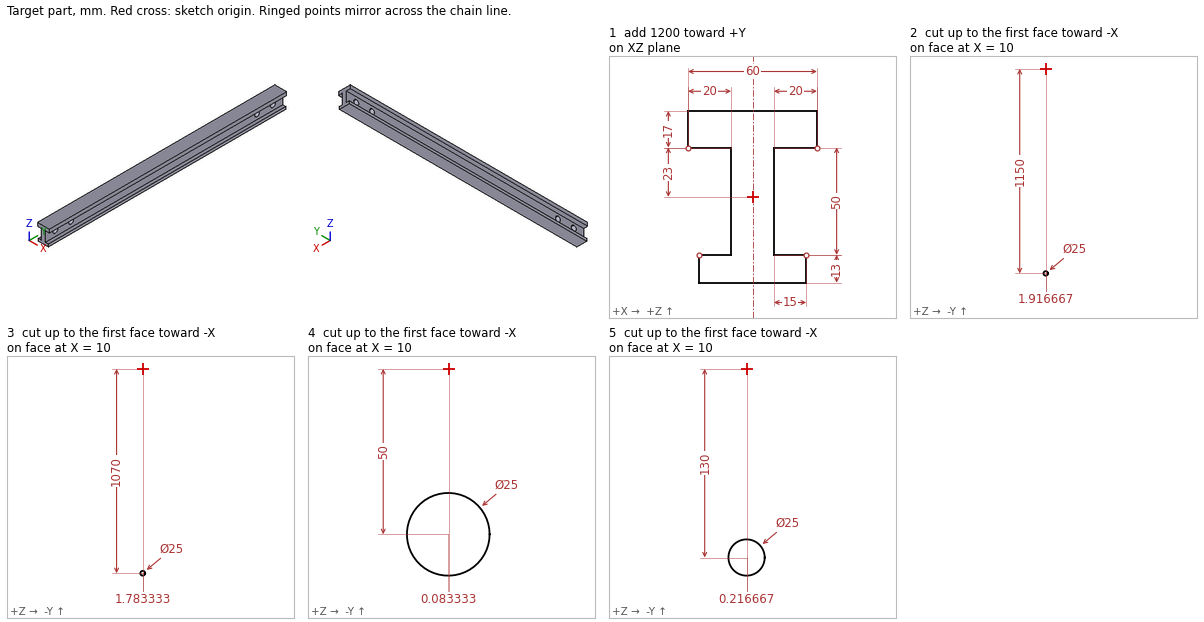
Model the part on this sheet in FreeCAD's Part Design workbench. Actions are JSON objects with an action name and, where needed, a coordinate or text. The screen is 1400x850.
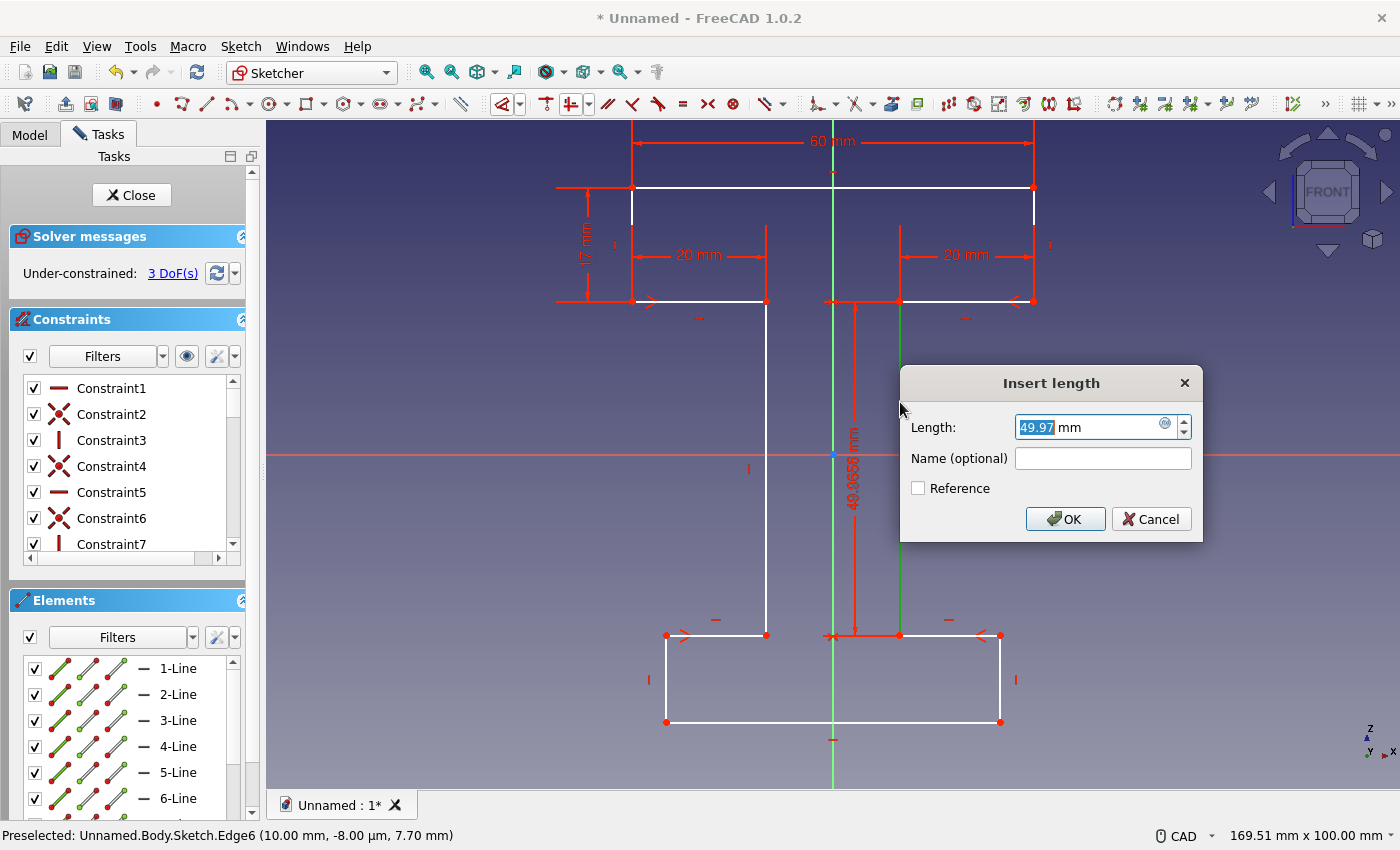
{"action": "type", "text": "50"}
{"action": "key", "text": "Return"}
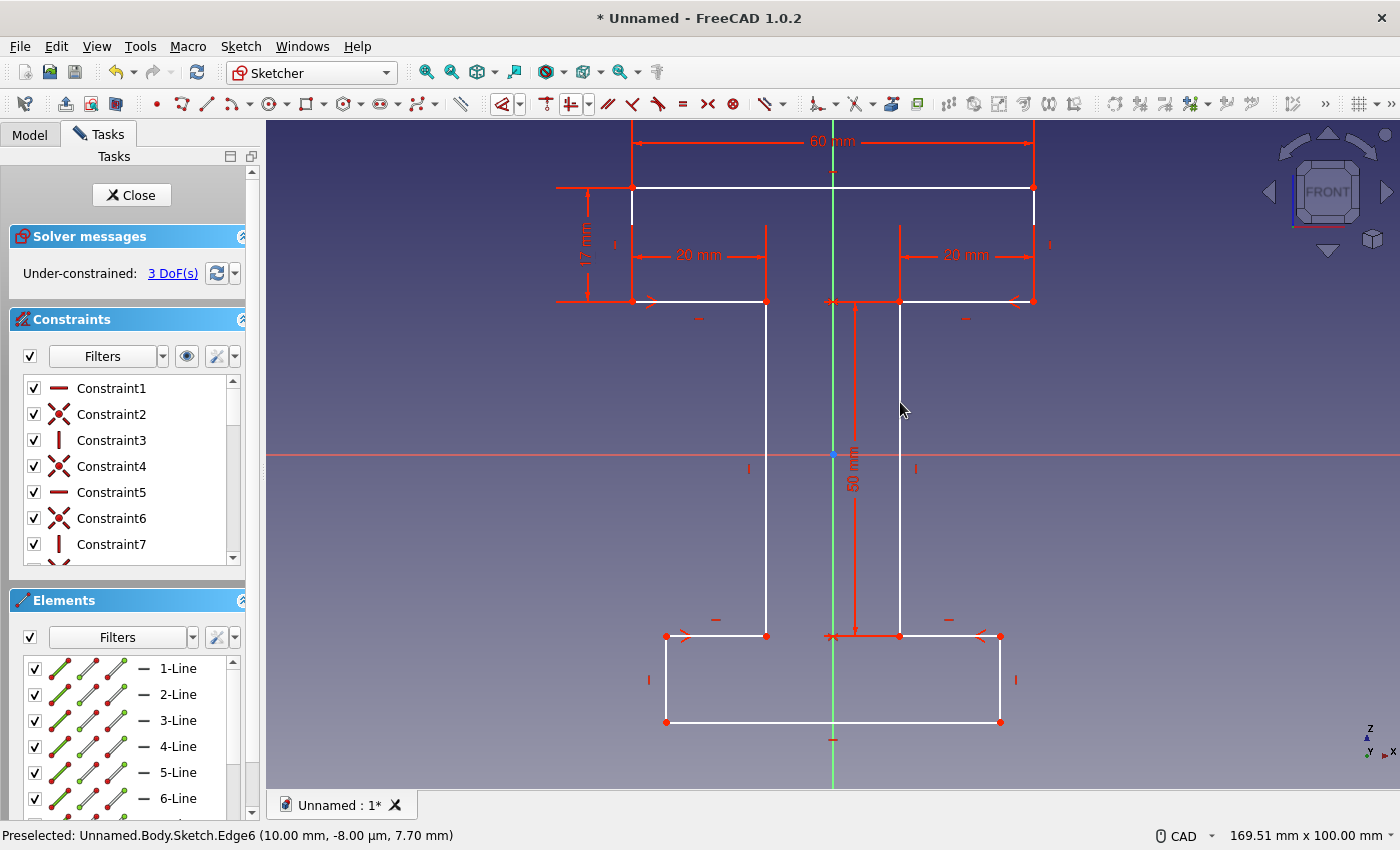
{"action": "left_click", "coordinate": [930, 636]}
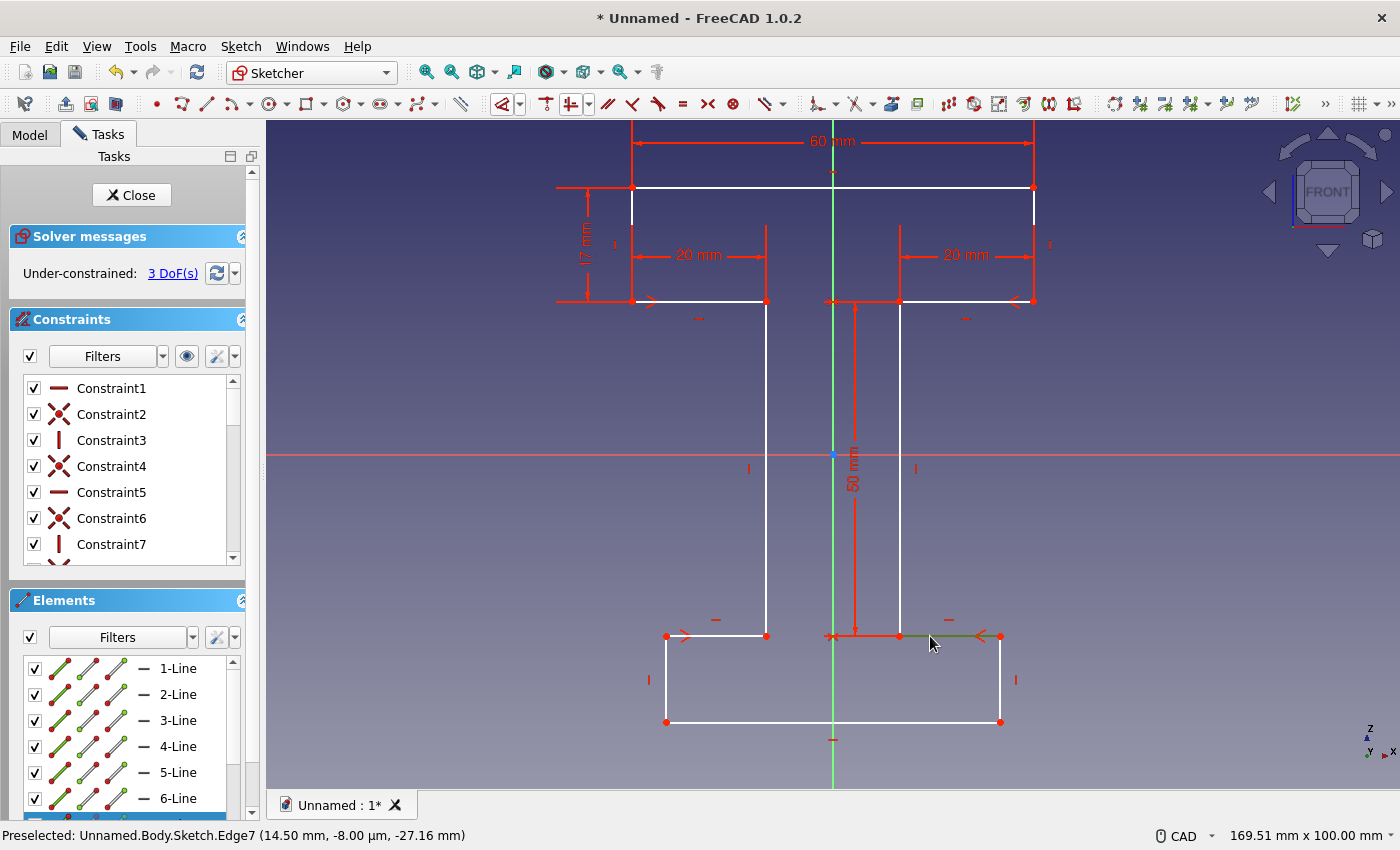
{"action": "key", "text": "l"}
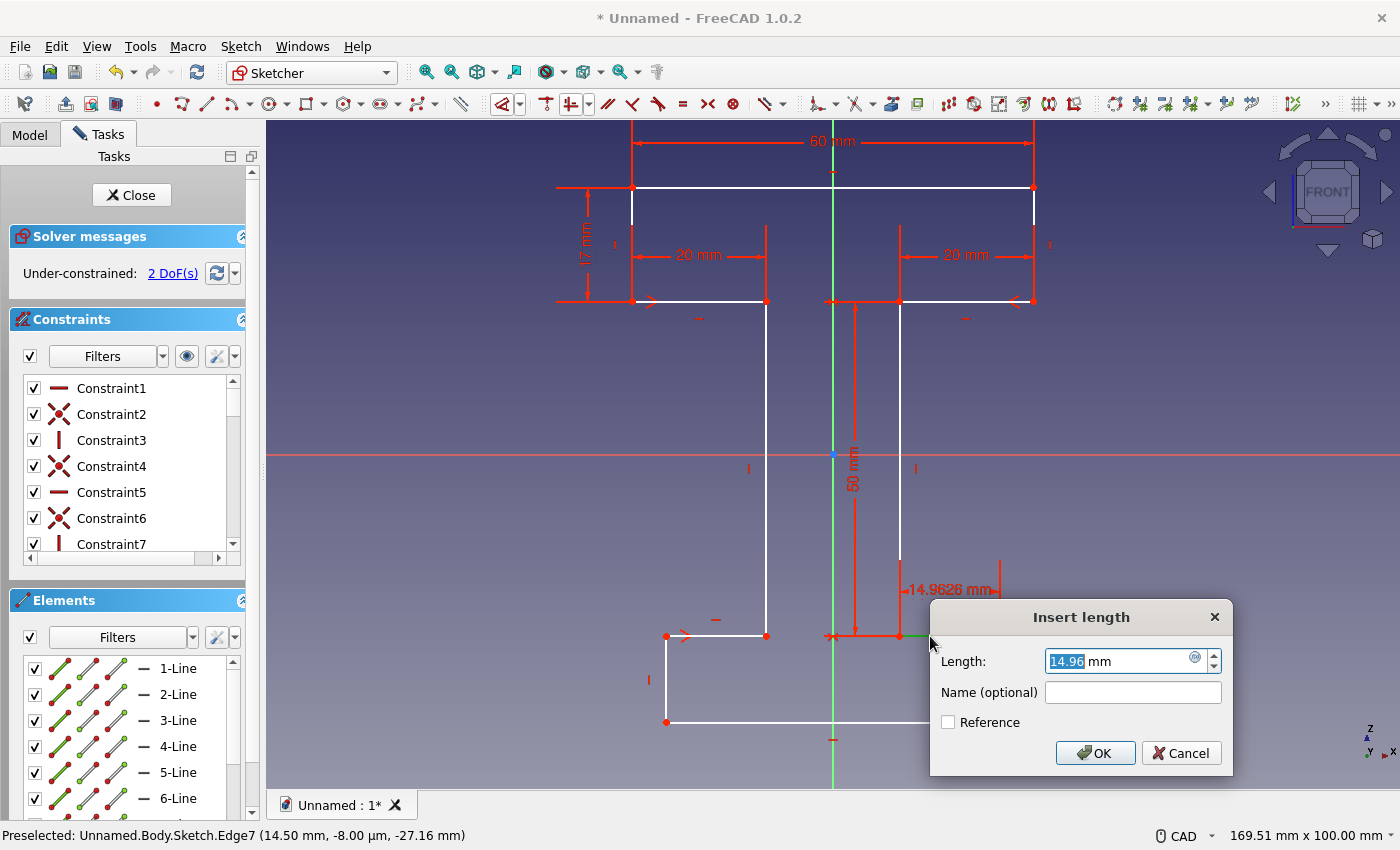
{"action": "type", "text": "15"}
{"action": "key", "text": "Return"}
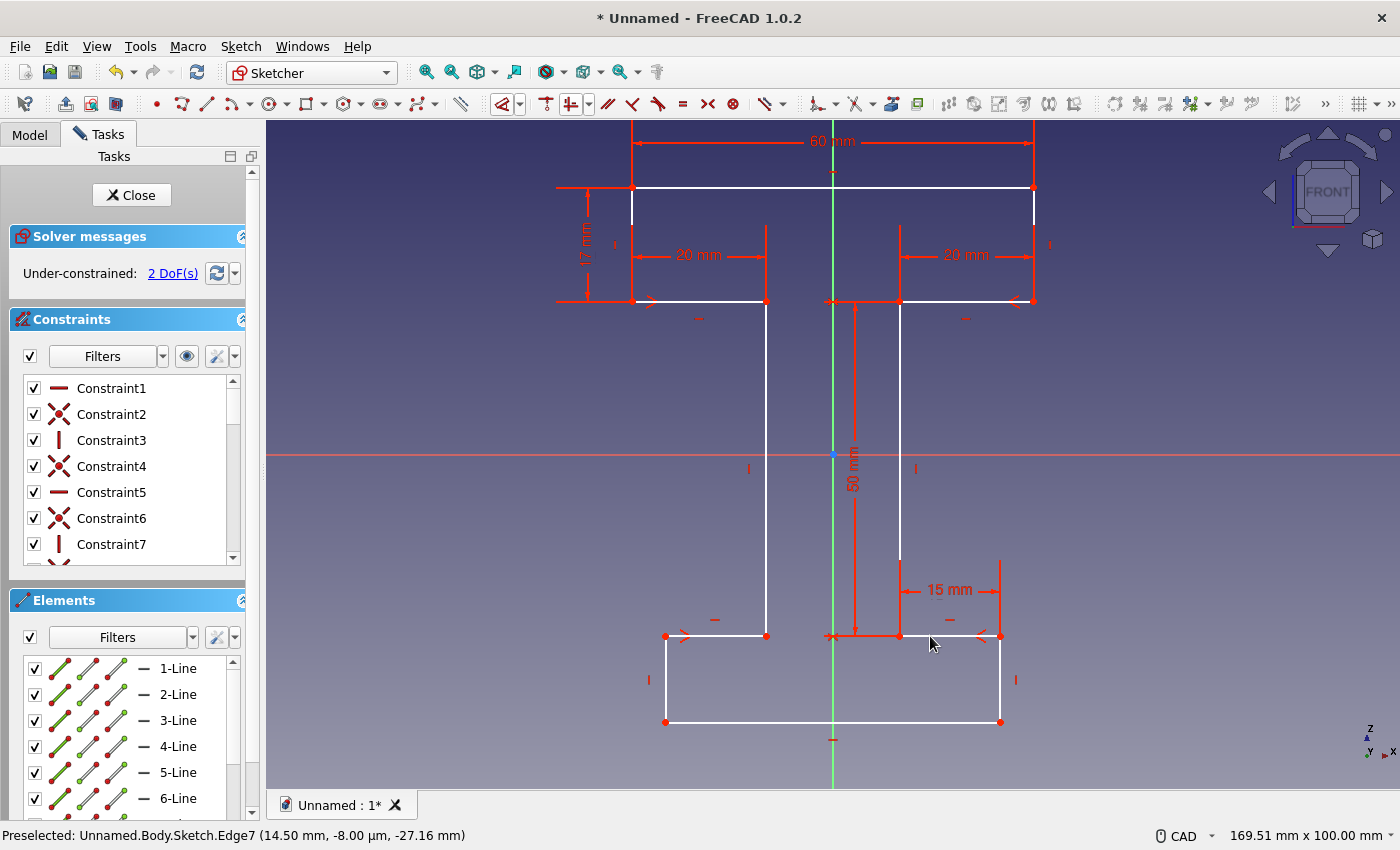
{"action": "left_click", "coordinate": [1000, 662]}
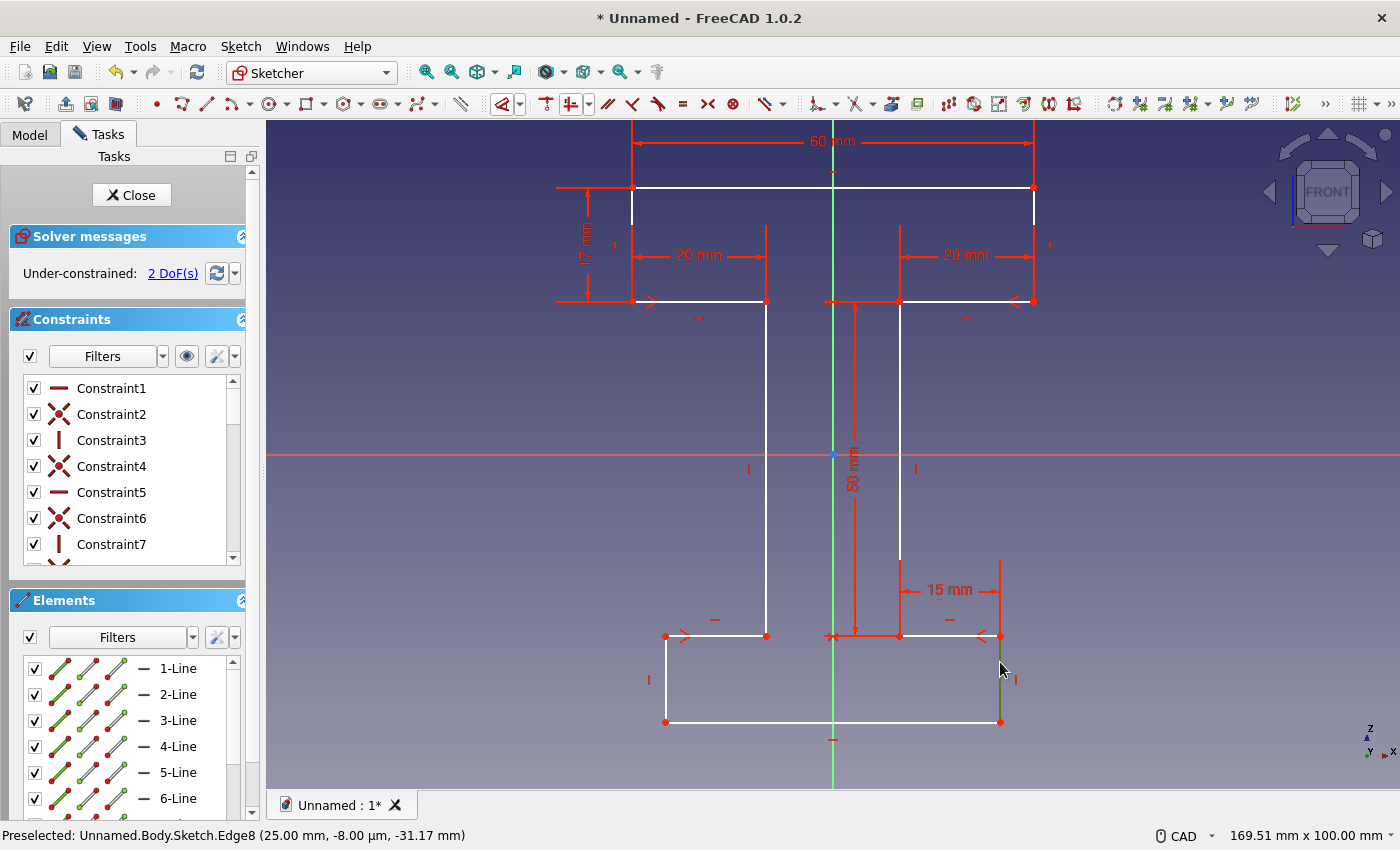
{"action": "left_click", "coordinate": [520, 104]}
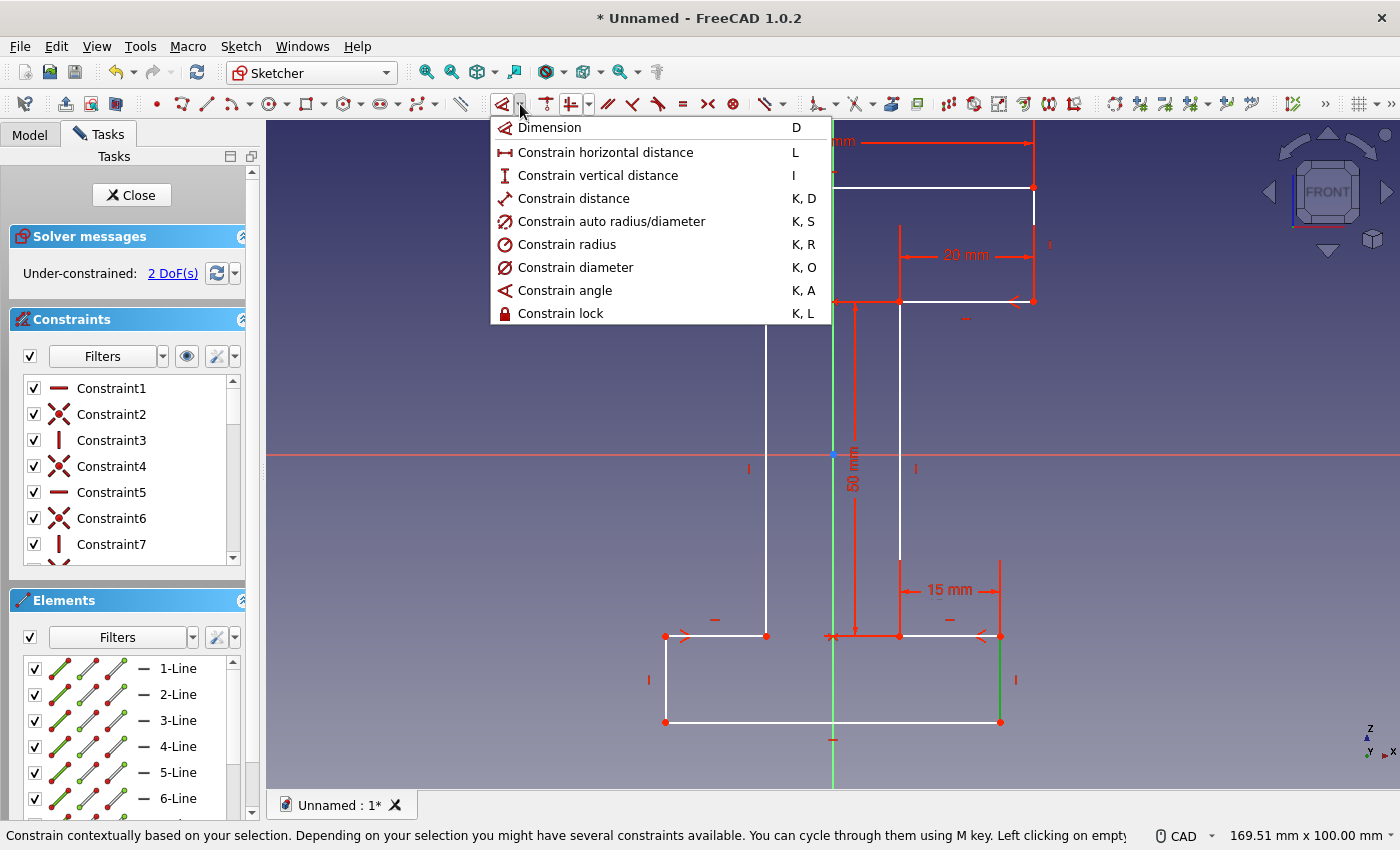
{"action": "left_click", "coordinate": [661, 176]}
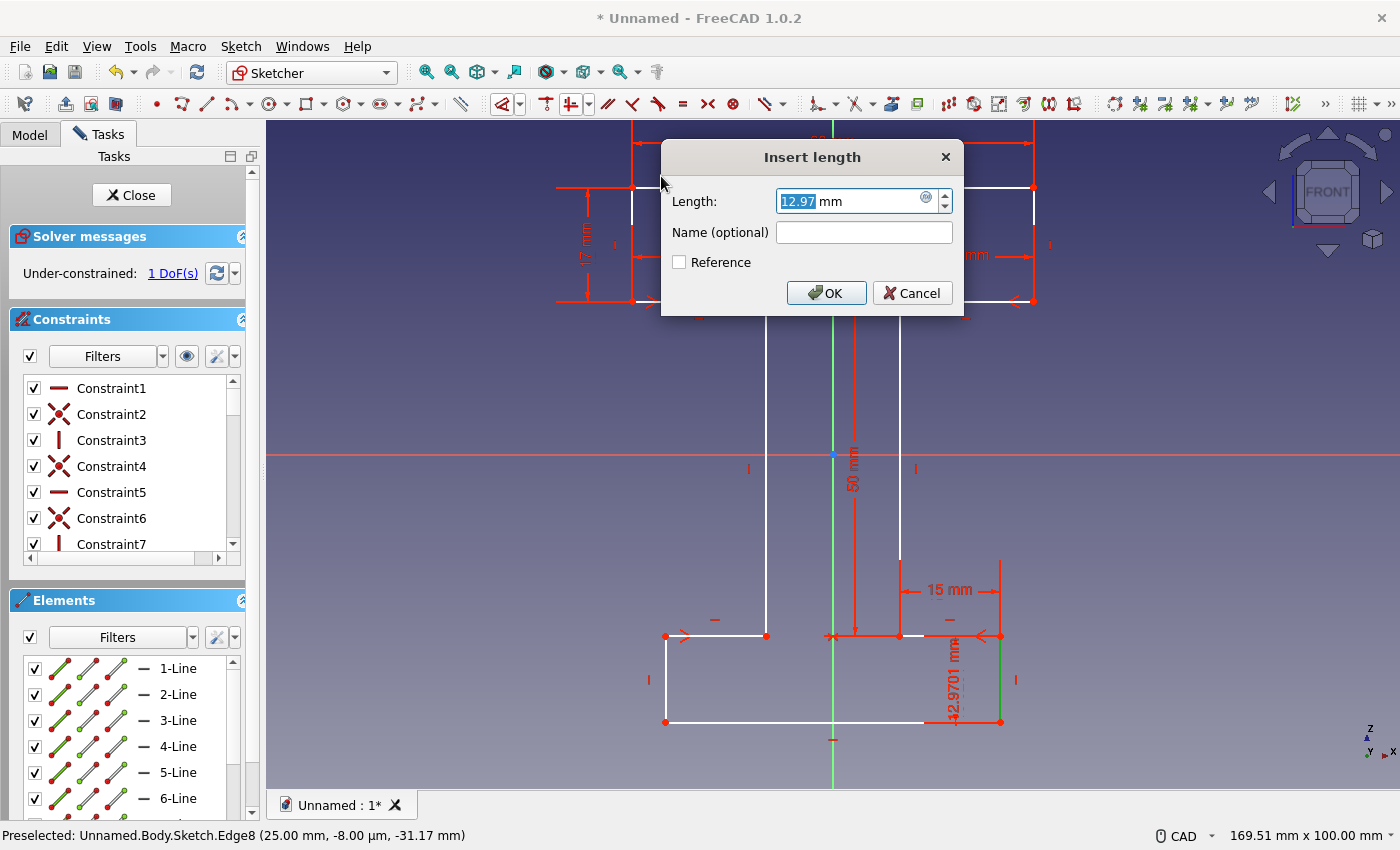
{"action": "type", "text": "13"}
{"action": "key", "text": "Return"}